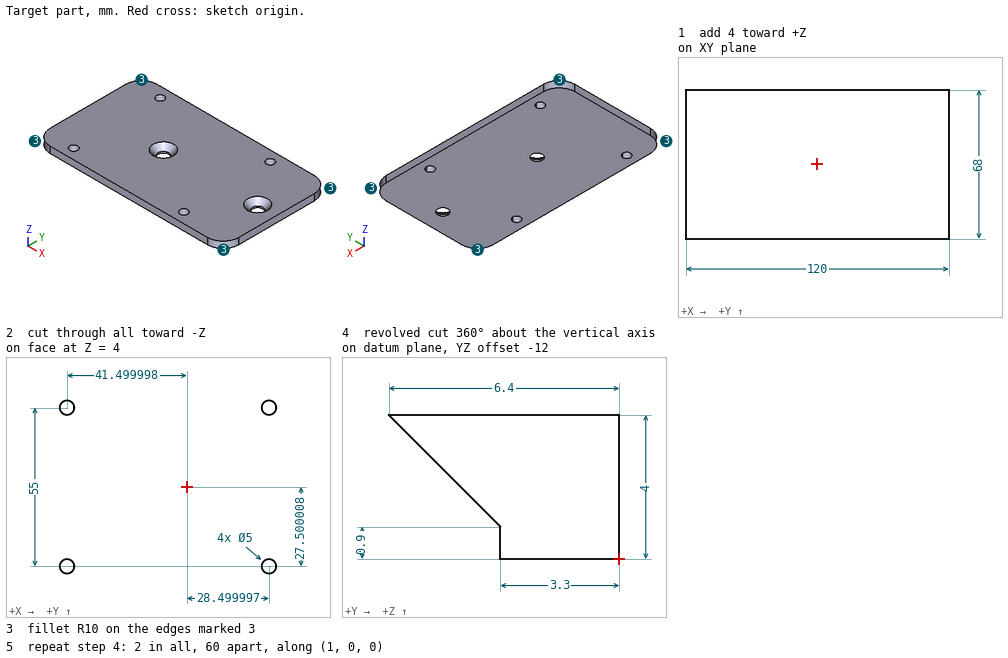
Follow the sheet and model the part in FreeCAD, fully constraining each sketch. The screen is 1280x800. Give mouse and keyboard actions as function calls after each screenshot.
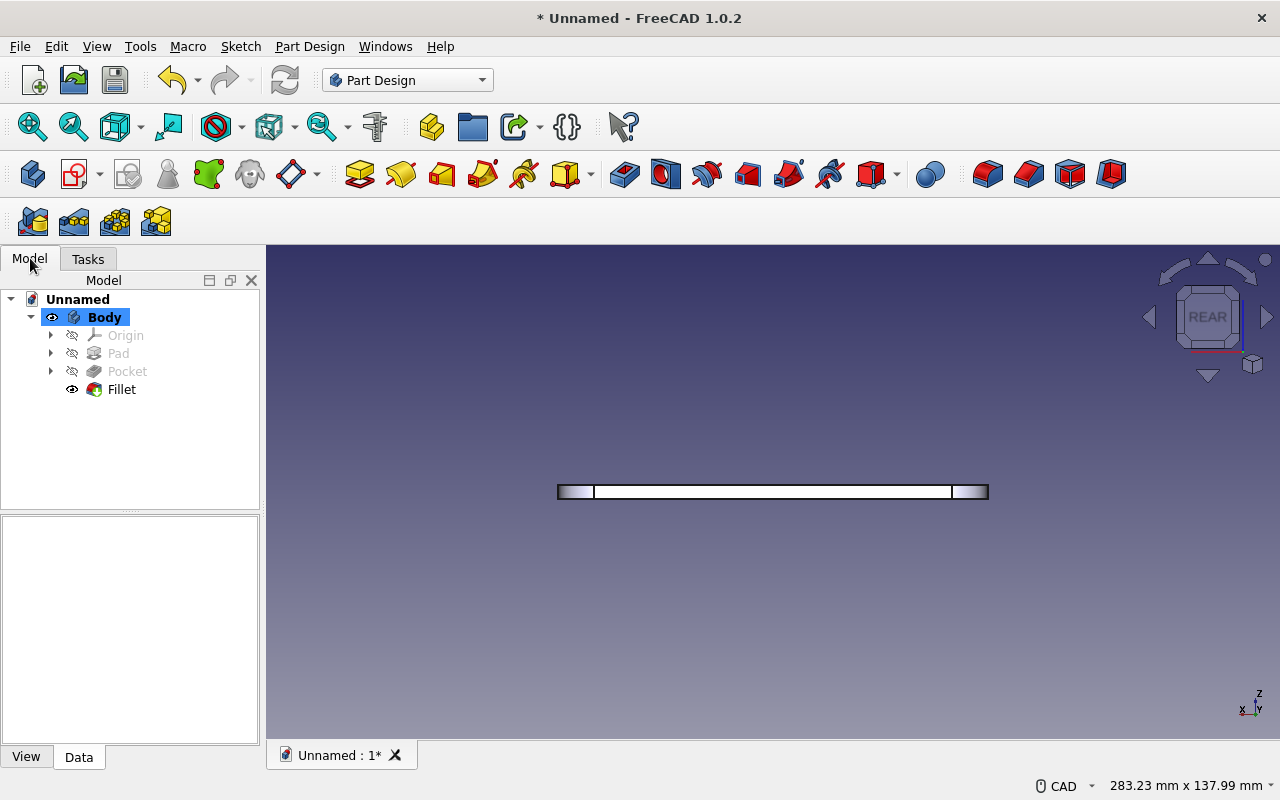
click(51, 335)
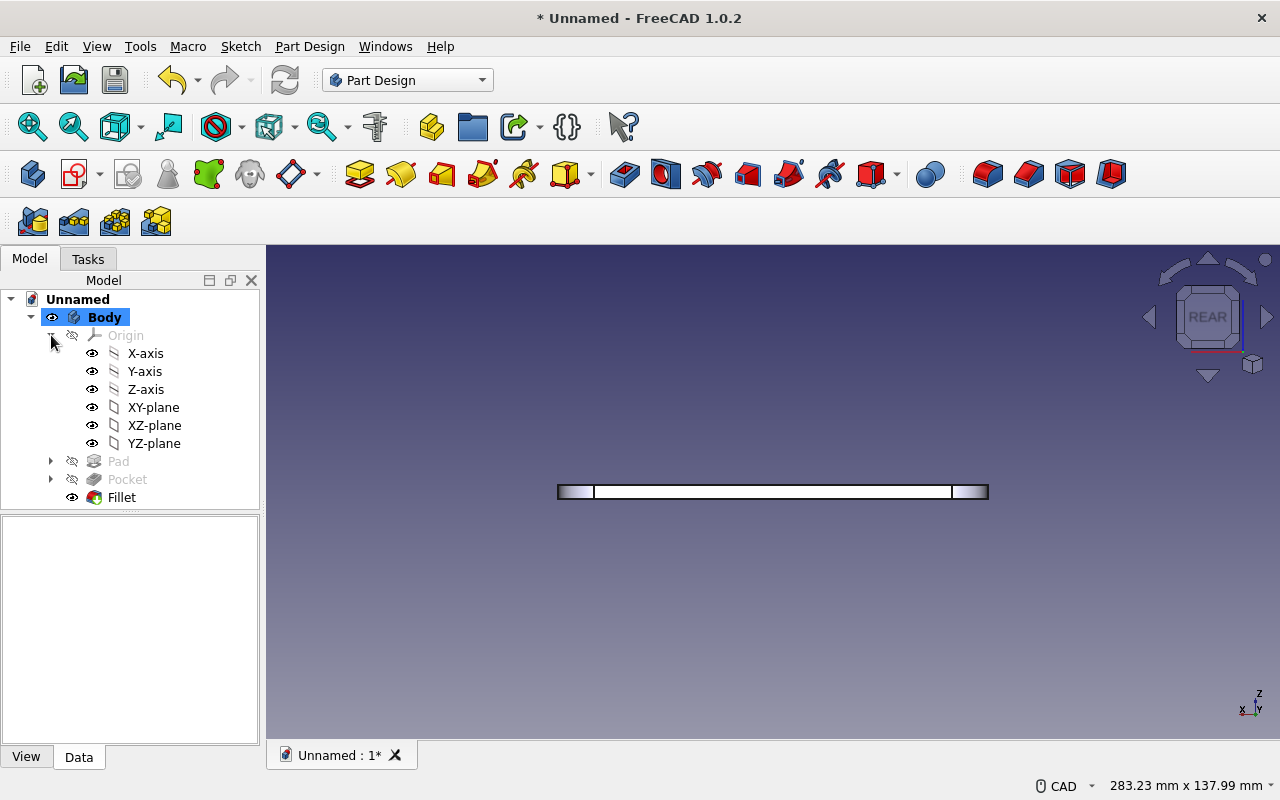
click(137, 443)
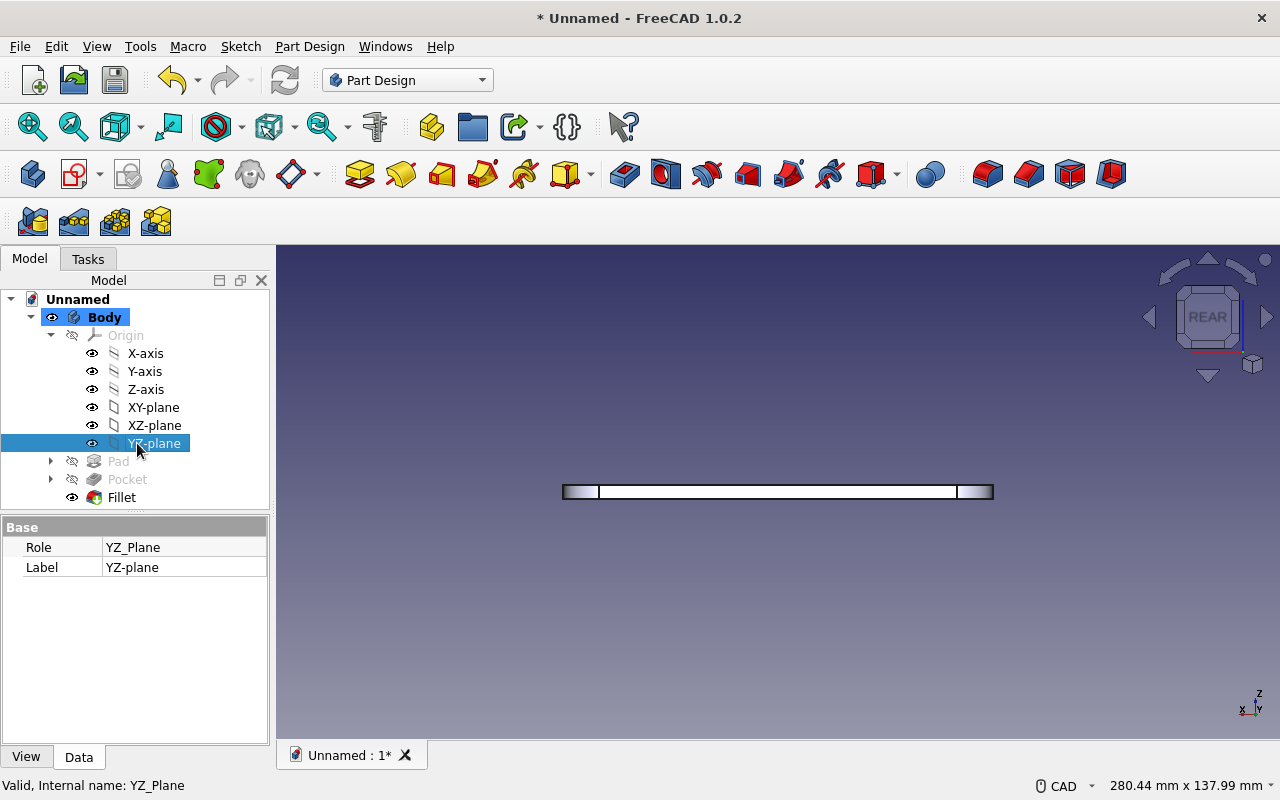
click(290, 174)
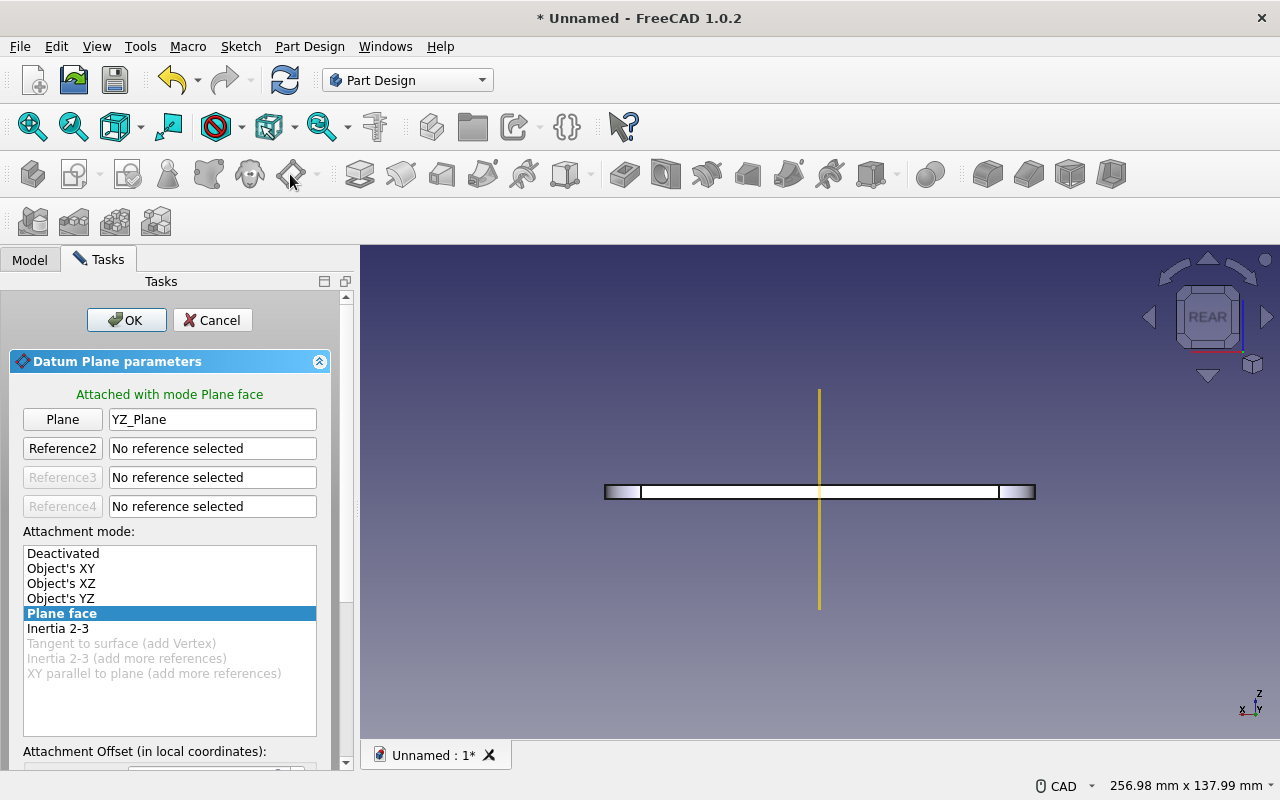
scroll(346, 530, down, 3)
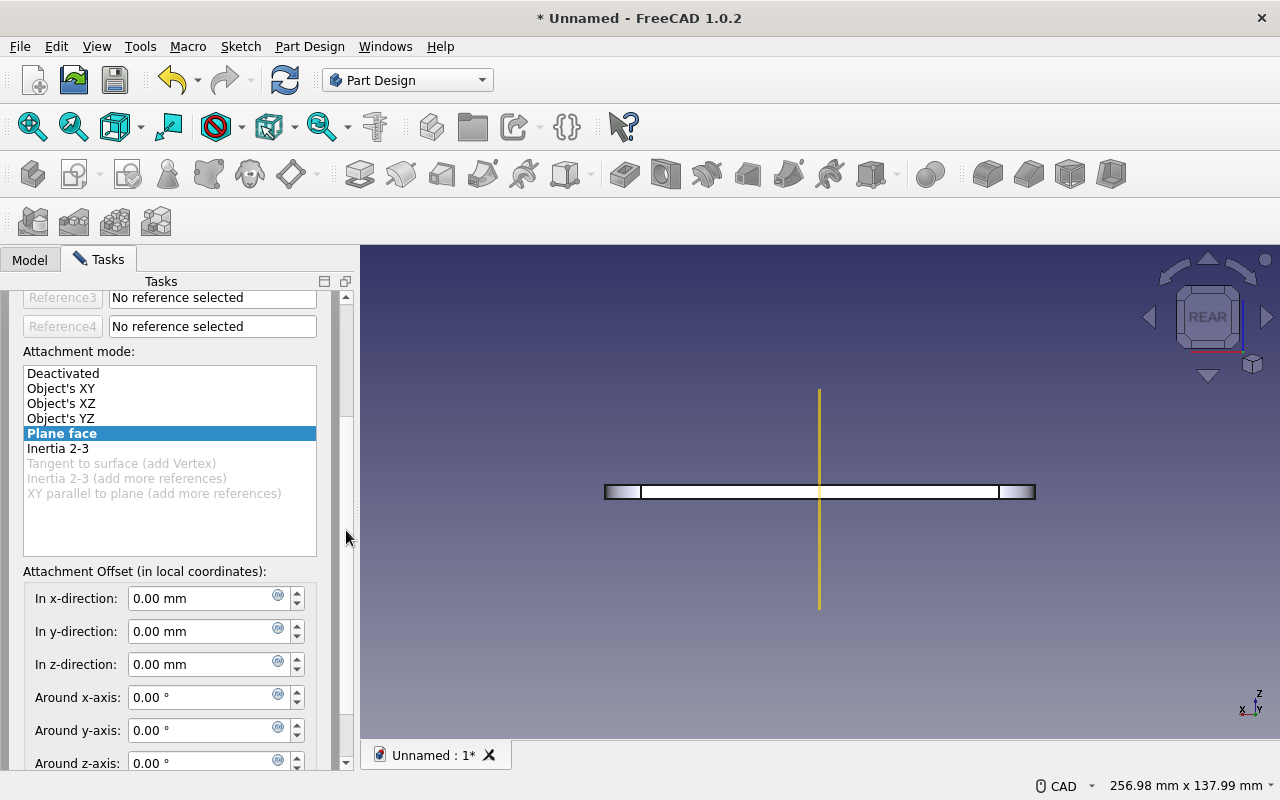
triple_click(210, 664)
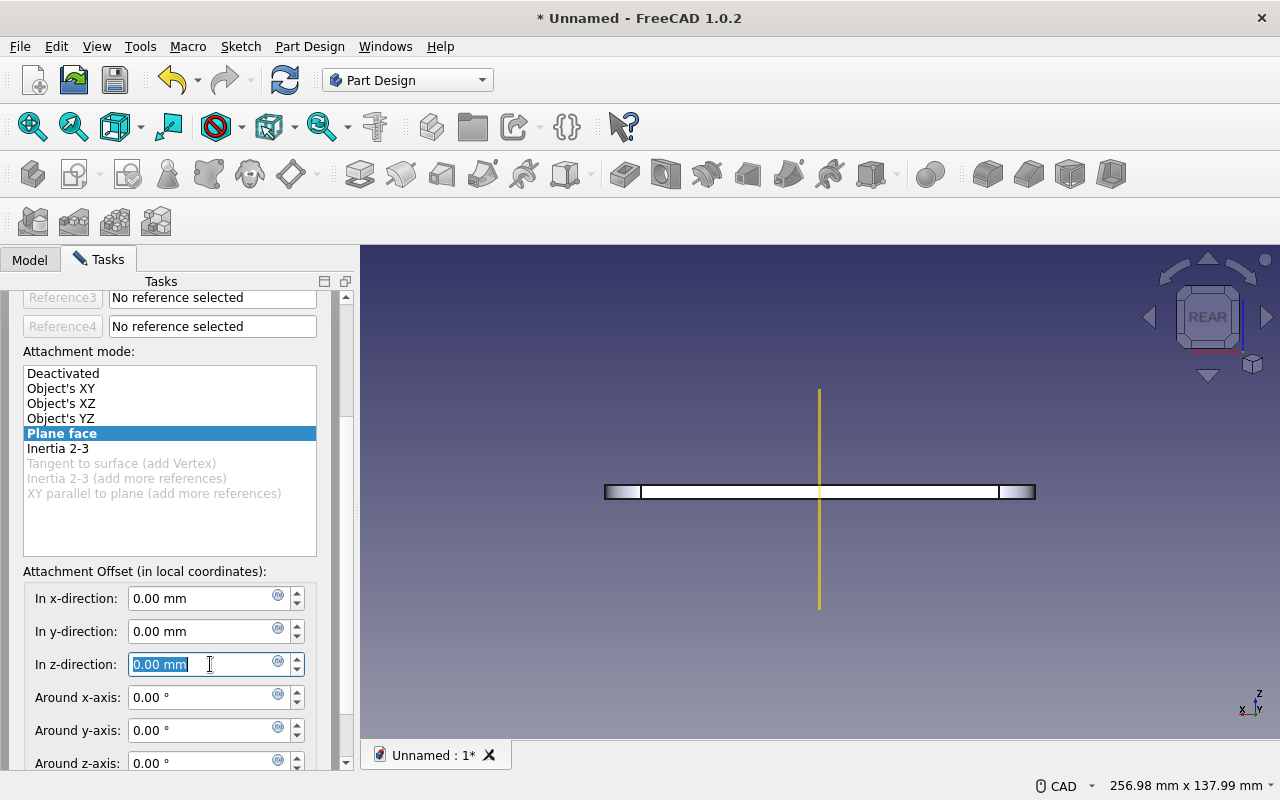
text(-12)
key(Tab)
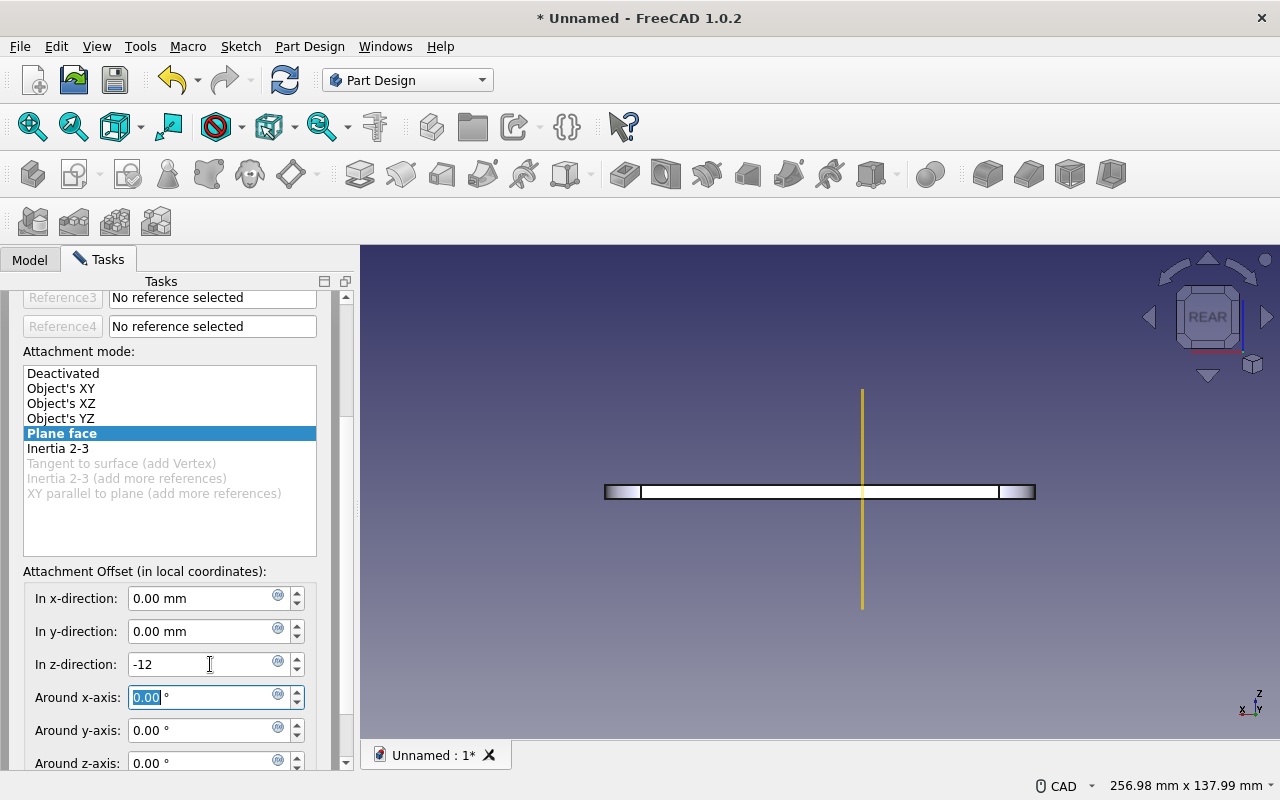
scroll(346, 530, up, 4)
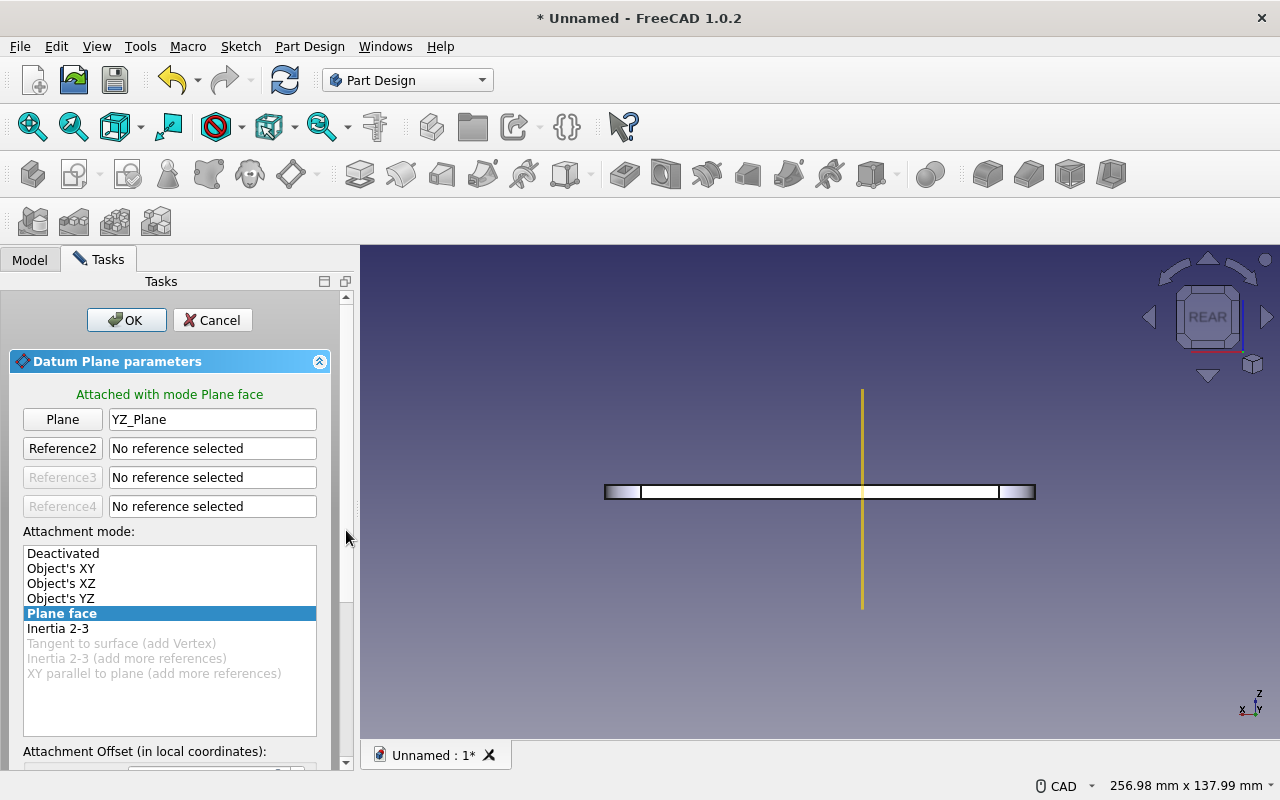
click(127, 320)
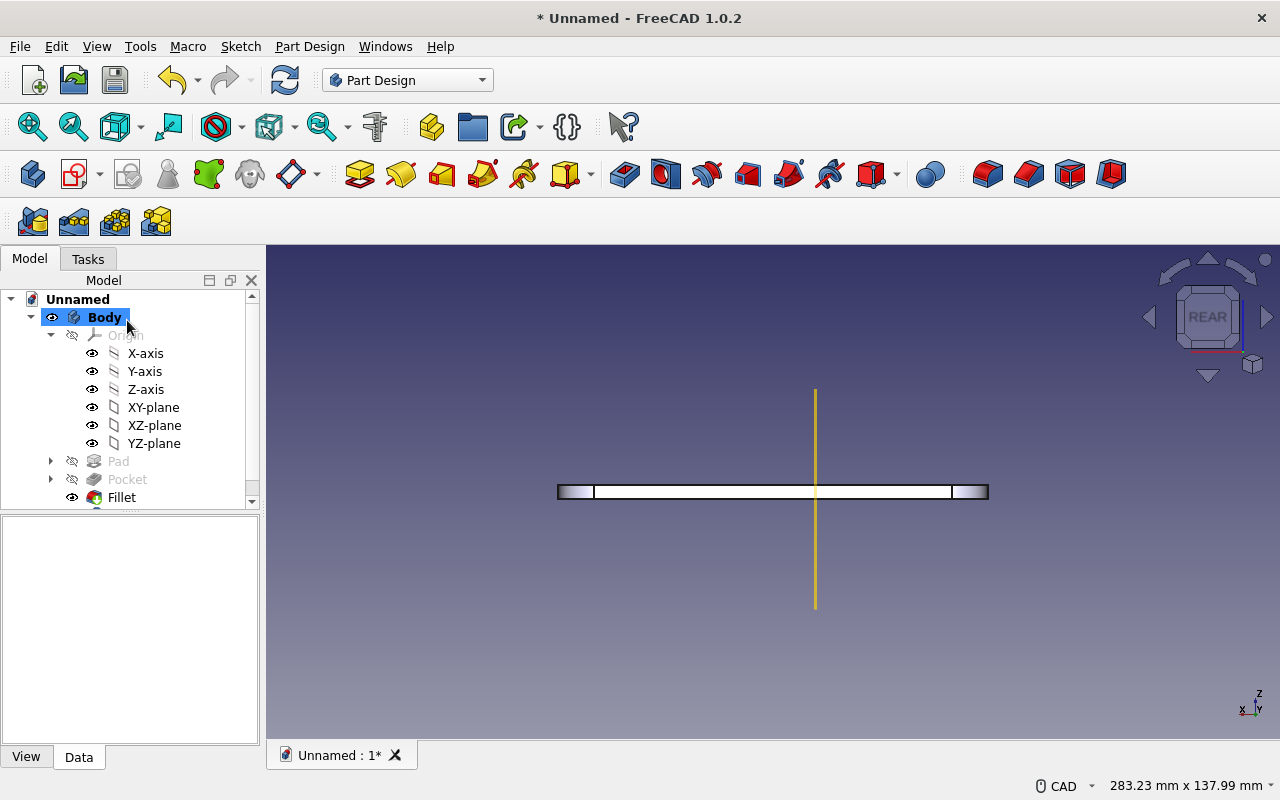
scroll(101, 403, down, 3)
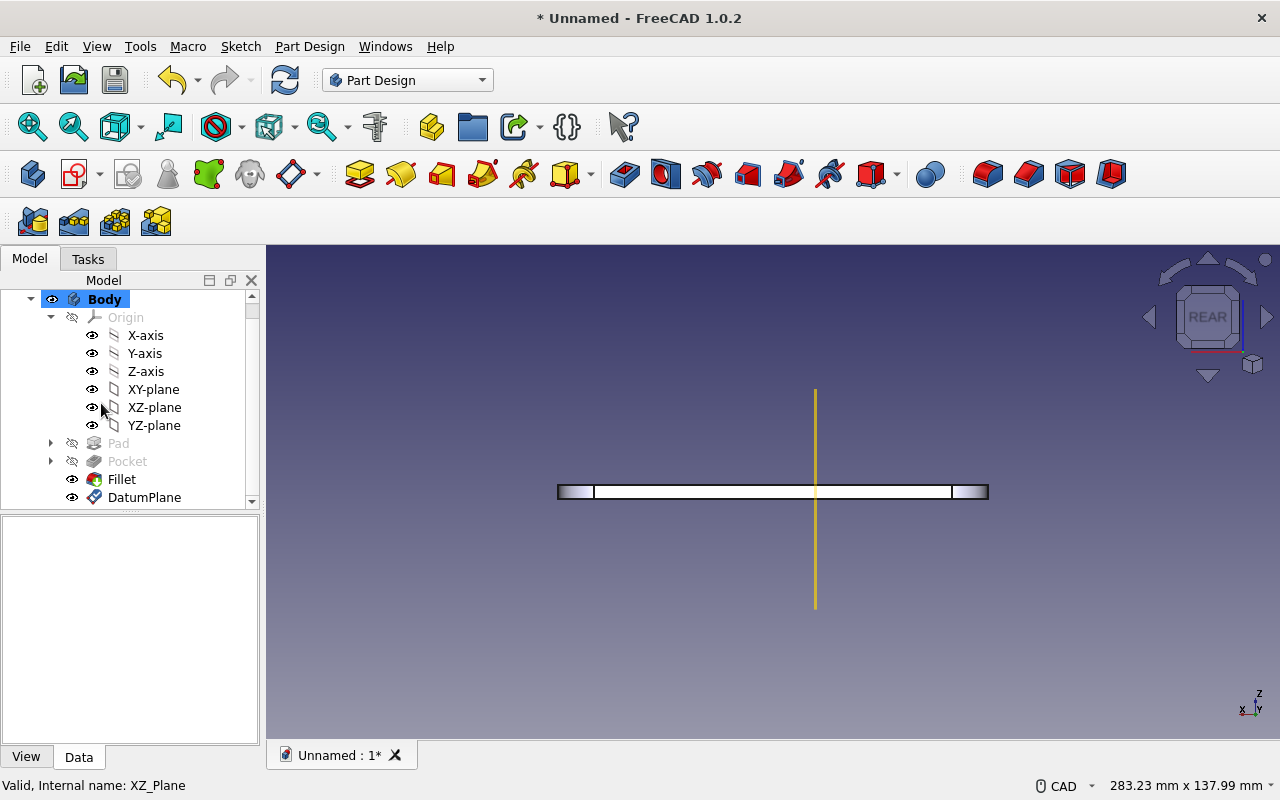
click(117, 497)